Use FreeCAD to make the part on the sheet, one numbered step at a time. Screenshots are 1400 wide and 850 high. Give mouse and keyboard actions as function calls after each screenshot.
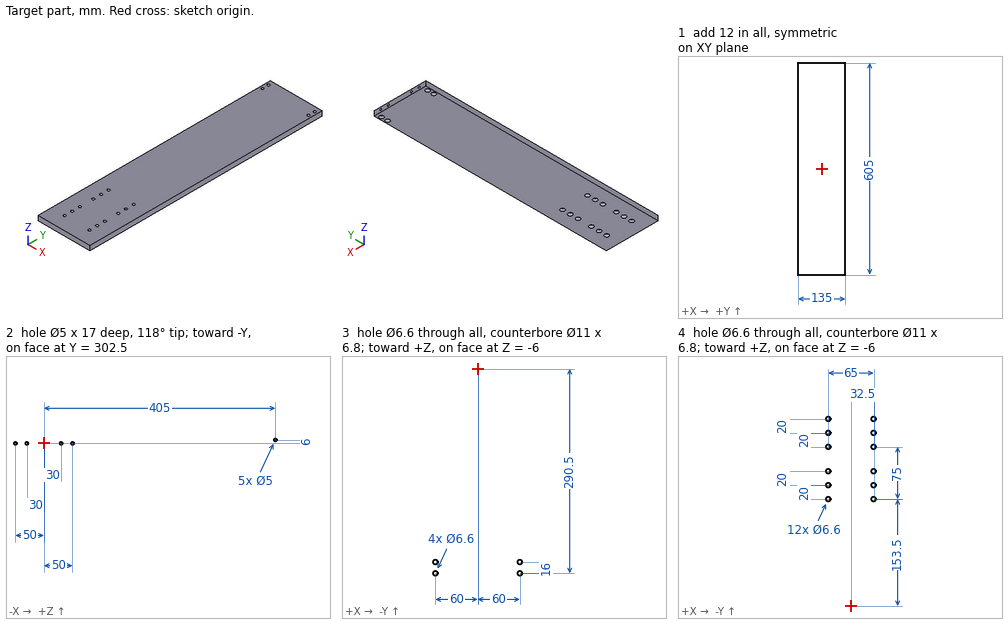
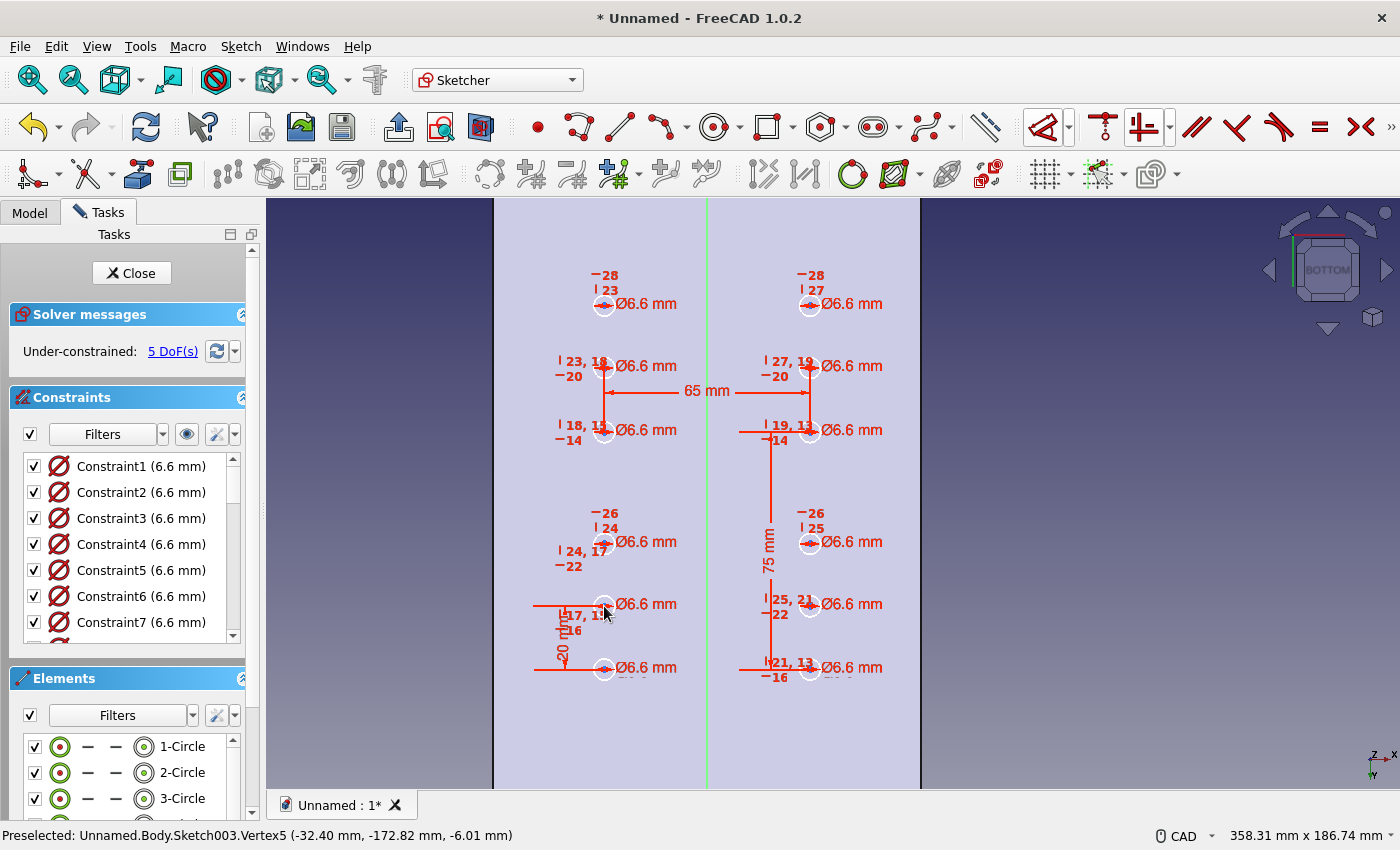
click(604, 432)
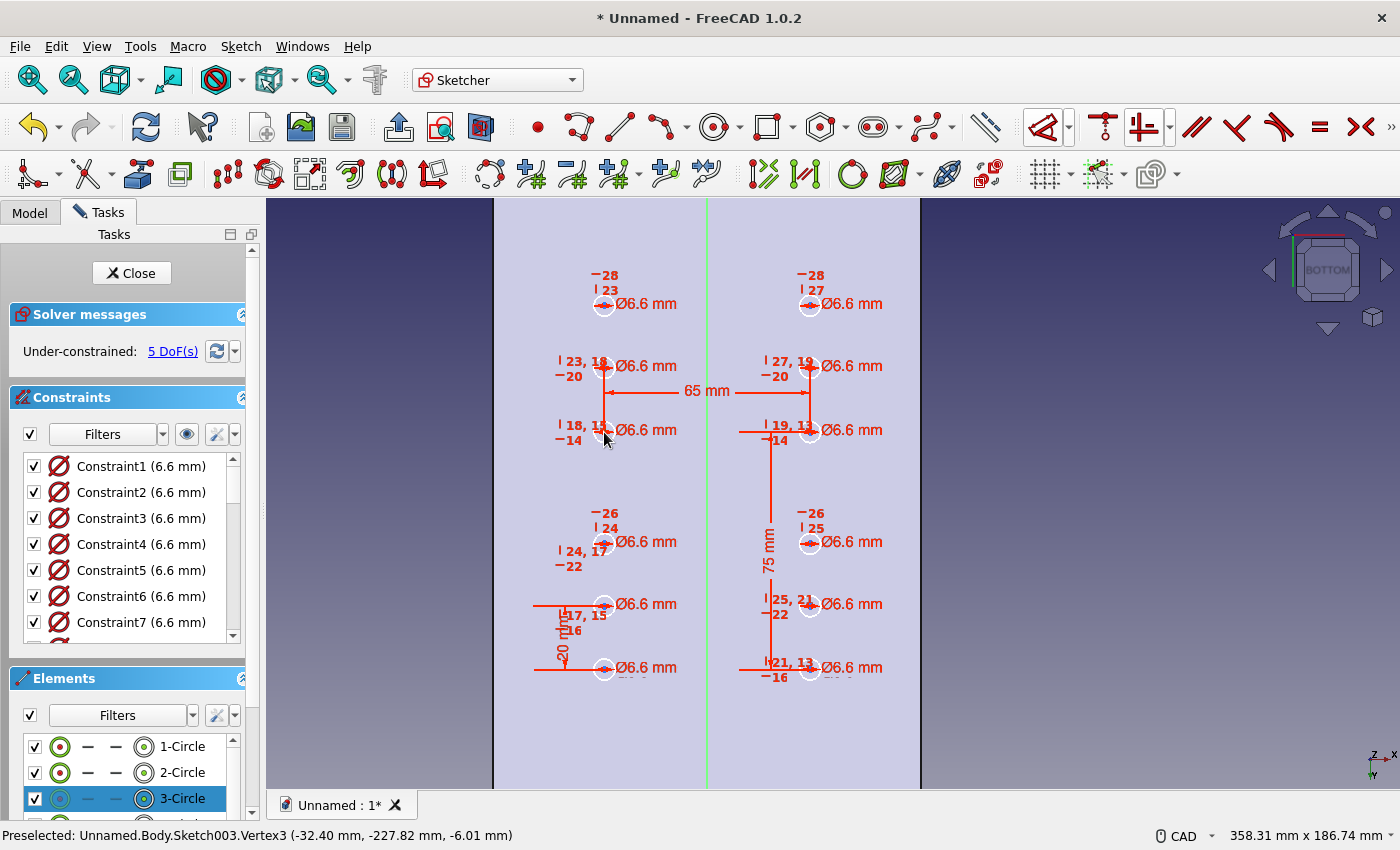
click(604, 368)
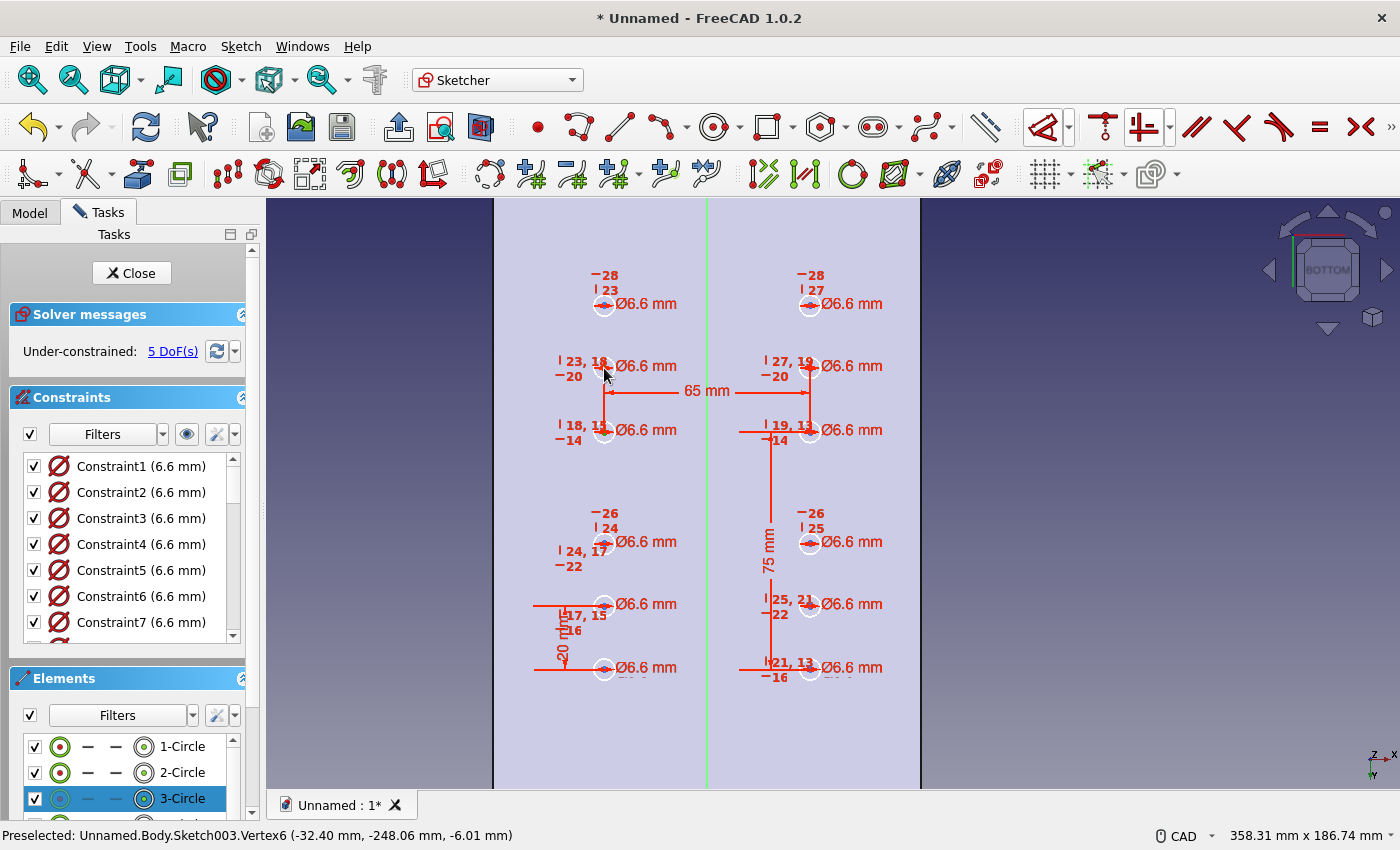
key(i)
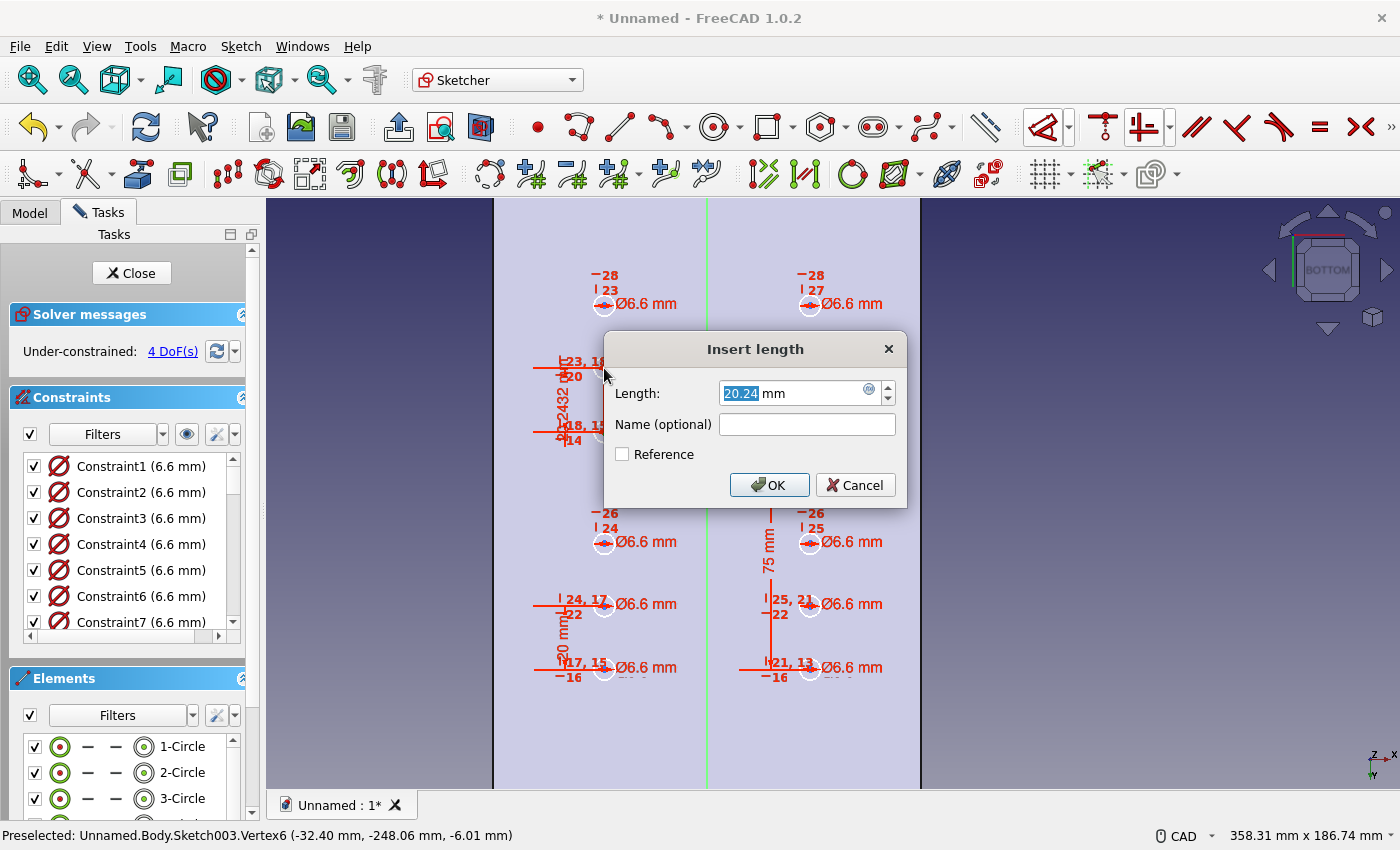
text(20)
key(Return)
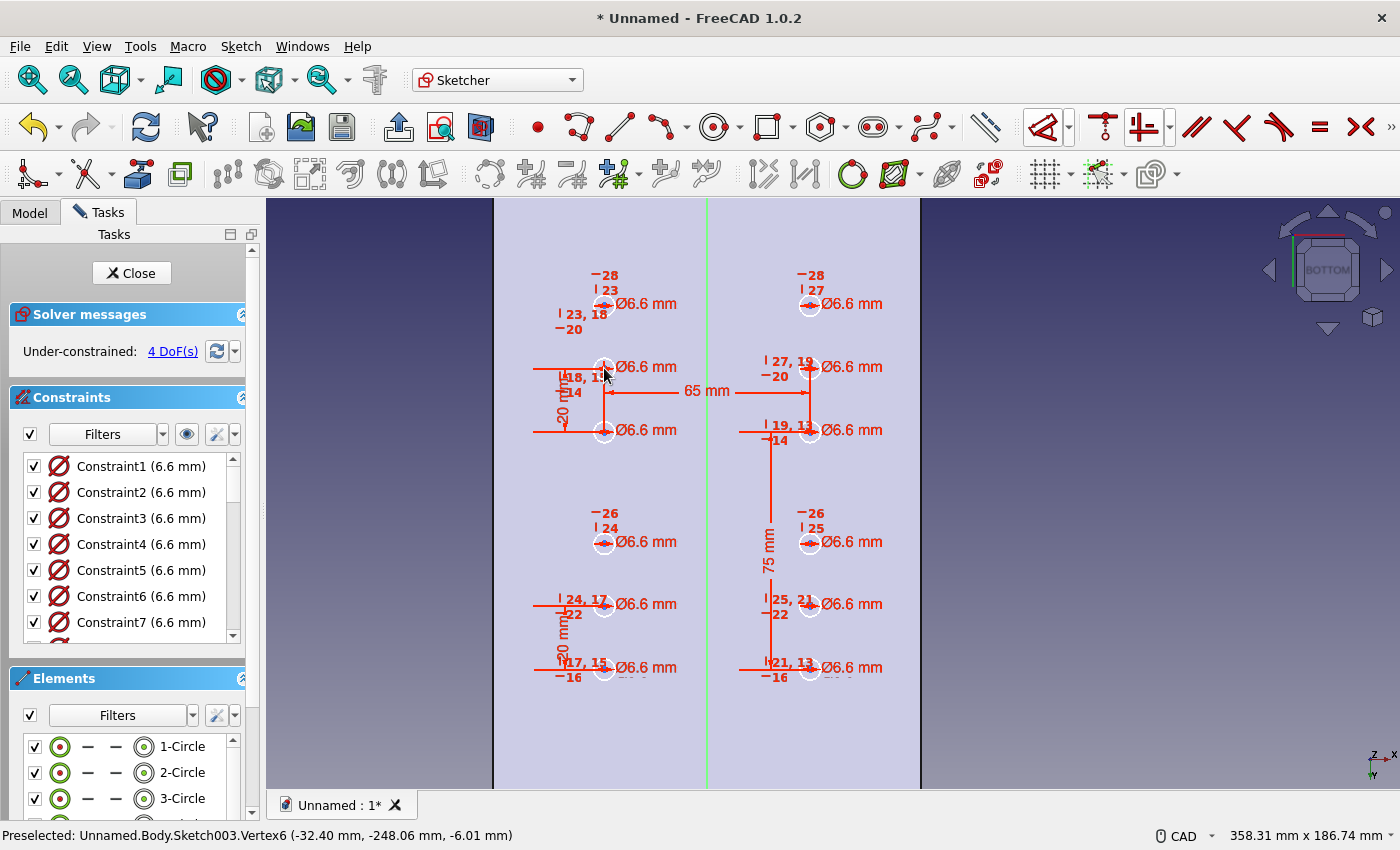
click(604, 369)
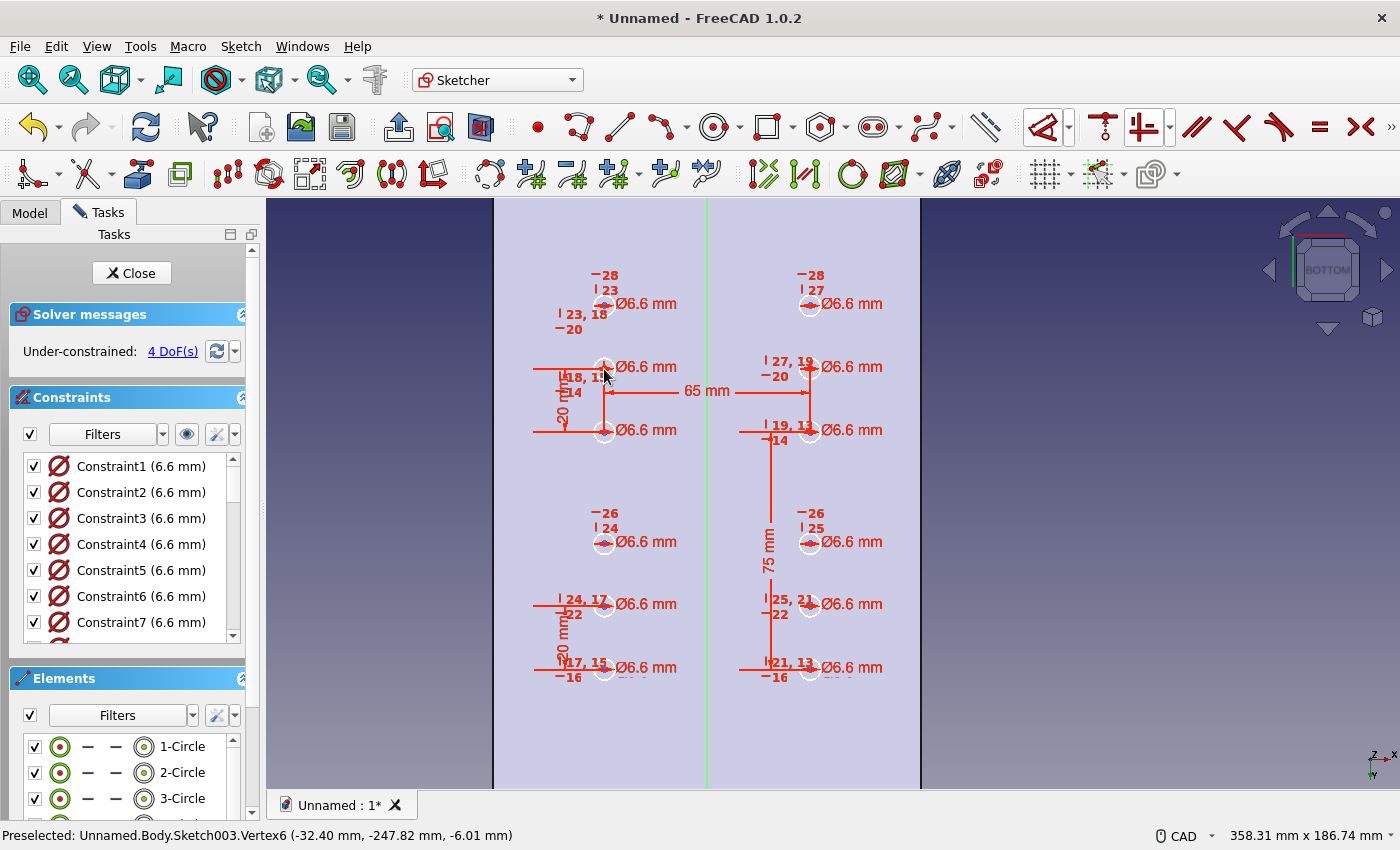
click(604, 306)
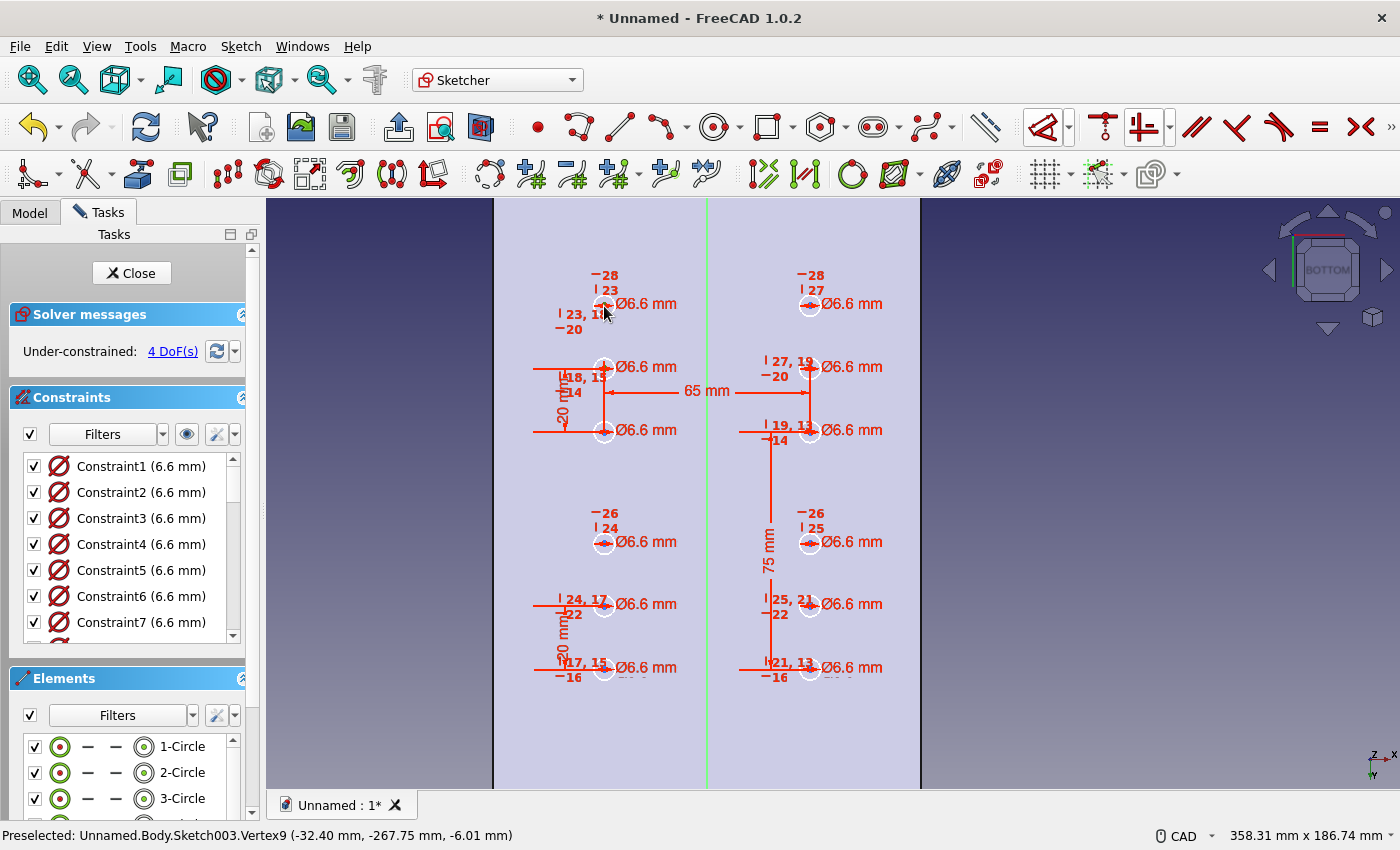
key(i)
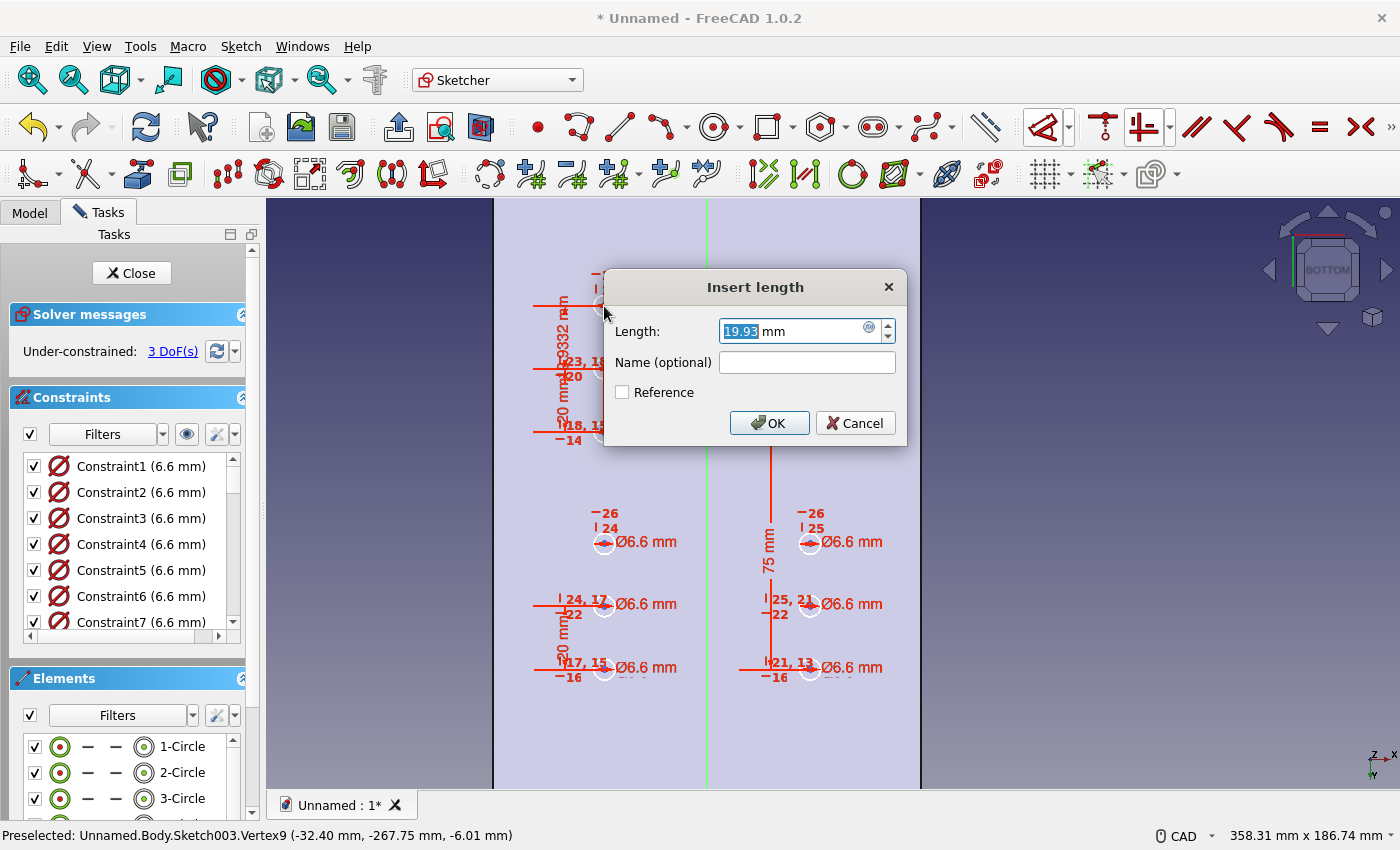
text(20)
key(Return)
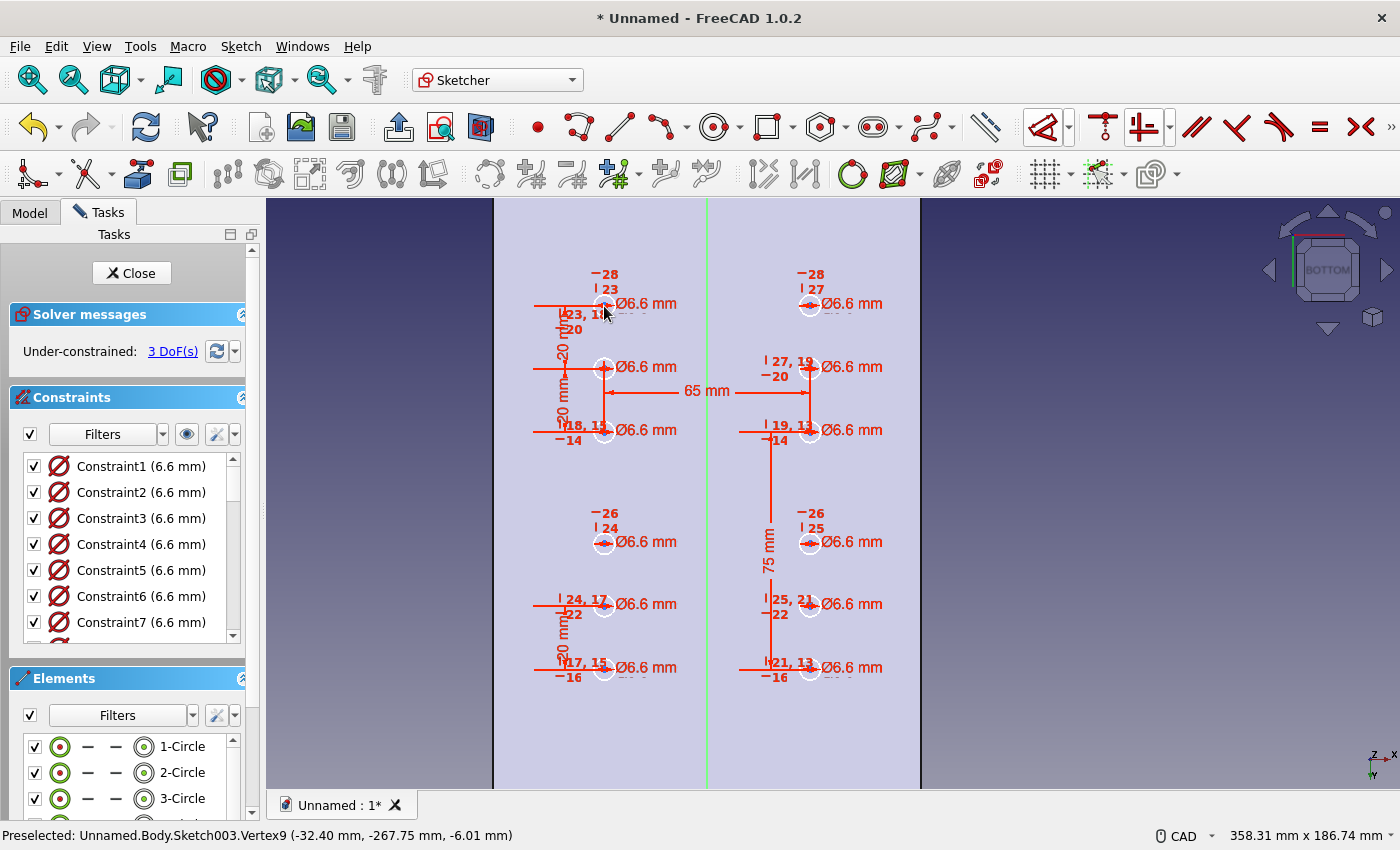
click(604, 606)